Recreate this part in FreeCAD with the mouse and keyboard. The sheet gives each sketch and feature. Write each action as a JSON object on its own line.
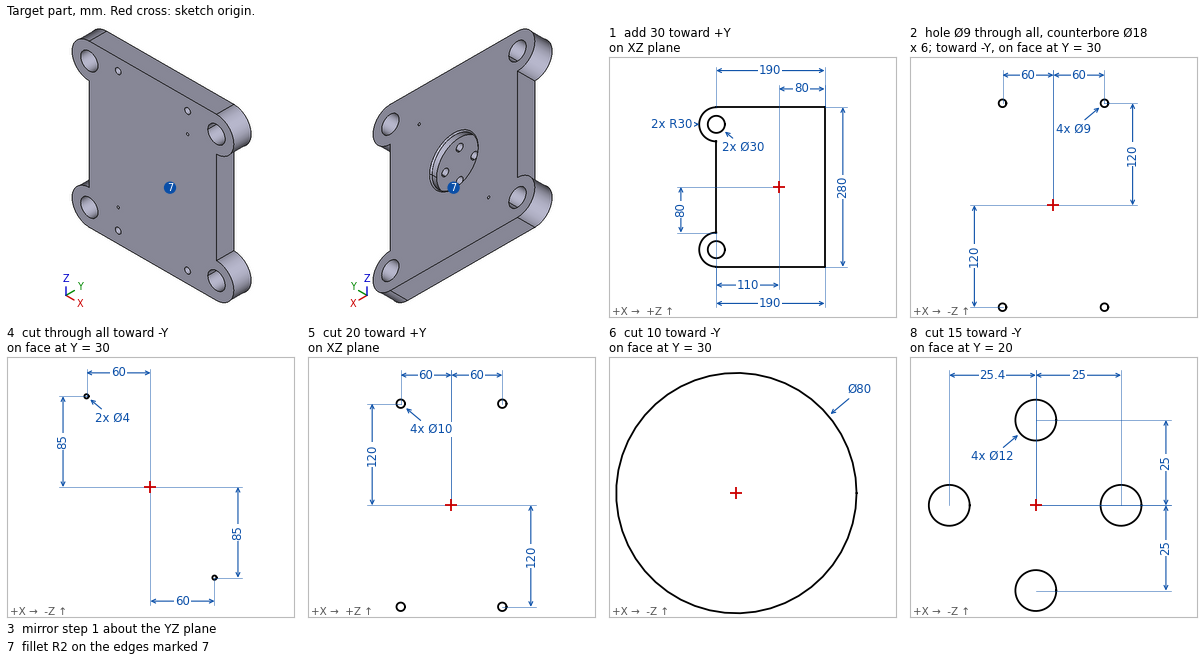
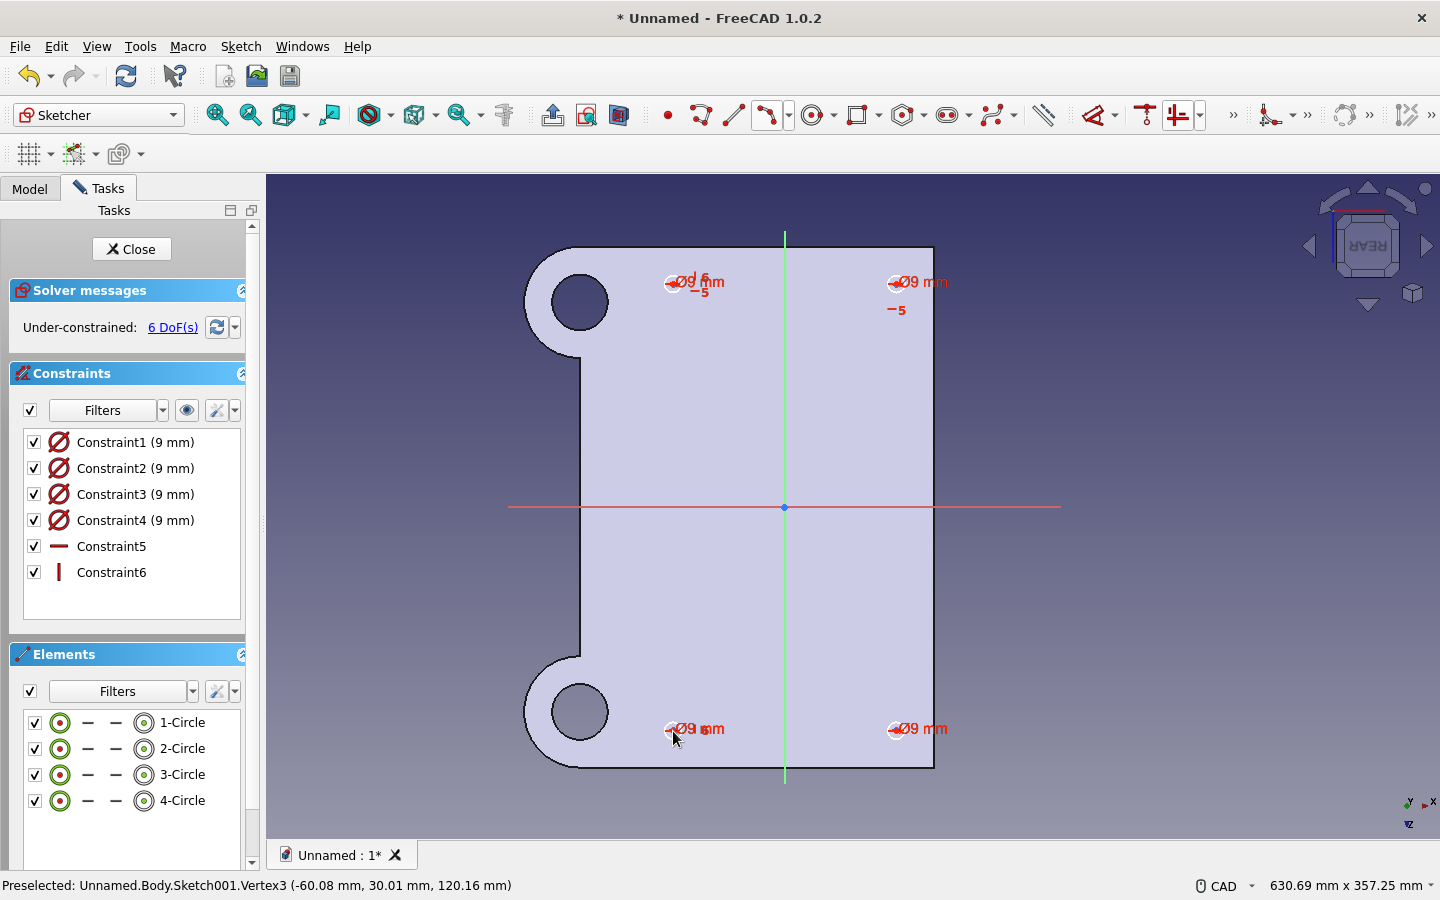
{"action": "left_click", "coordinate": [896, 284]}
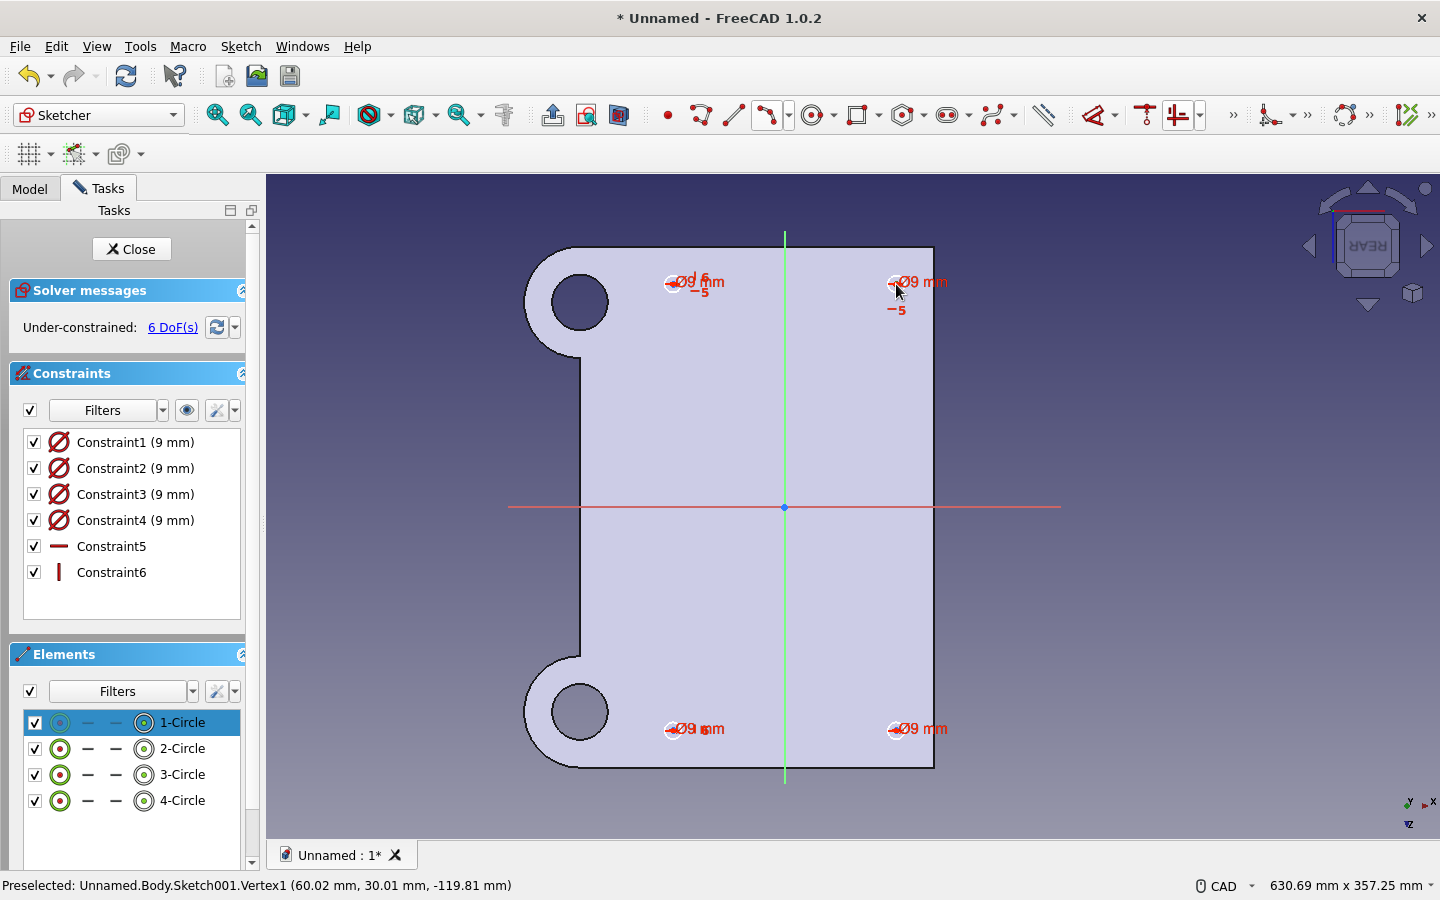
{"action": "left_click", "coordinate": [896, 731]}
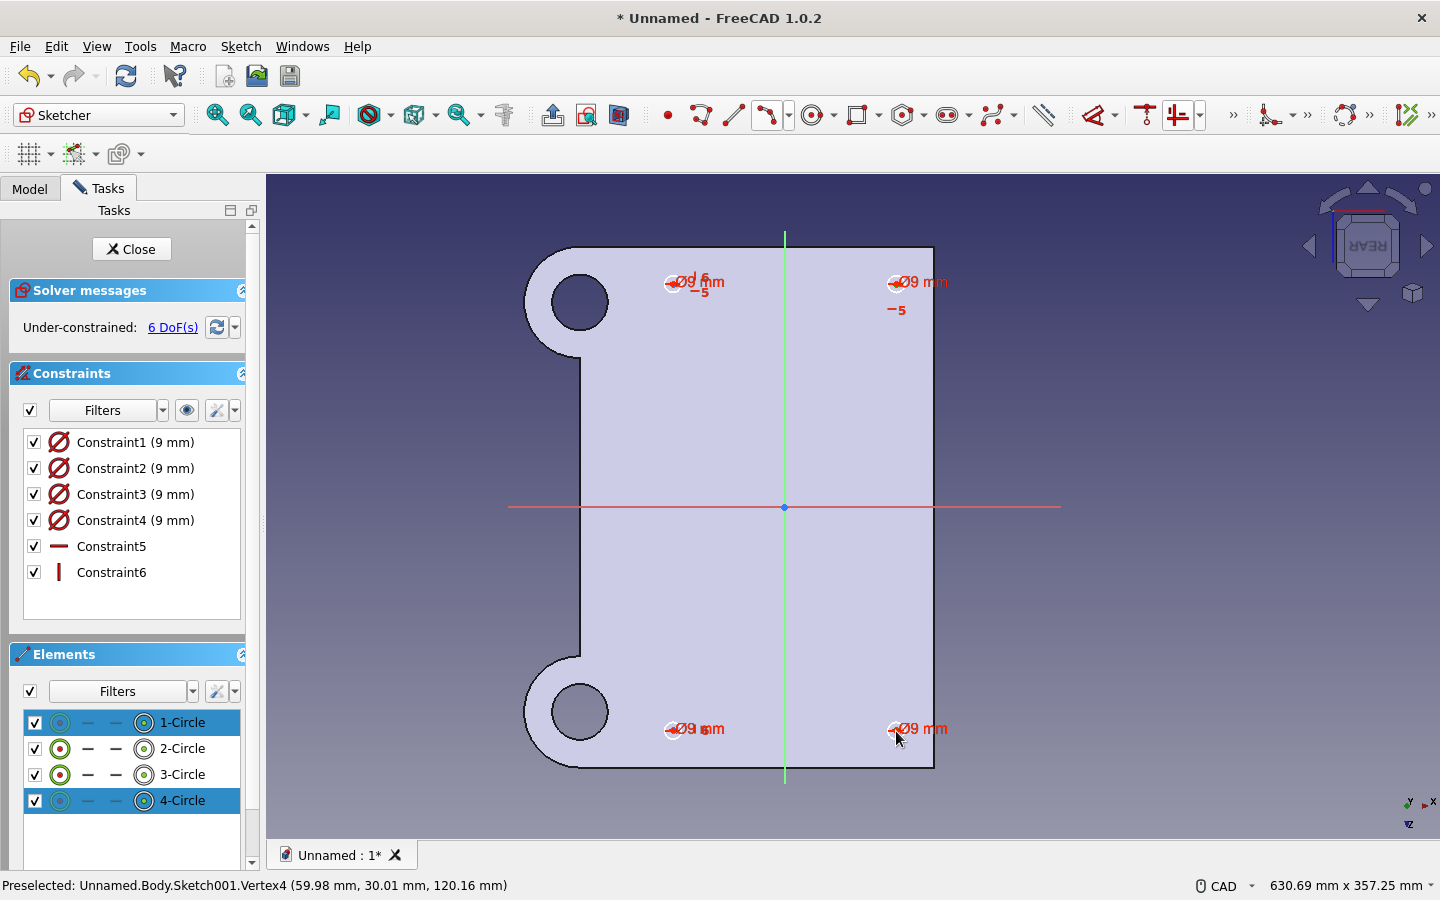
{"action": "left_click", "coordinate": [1200, 116]}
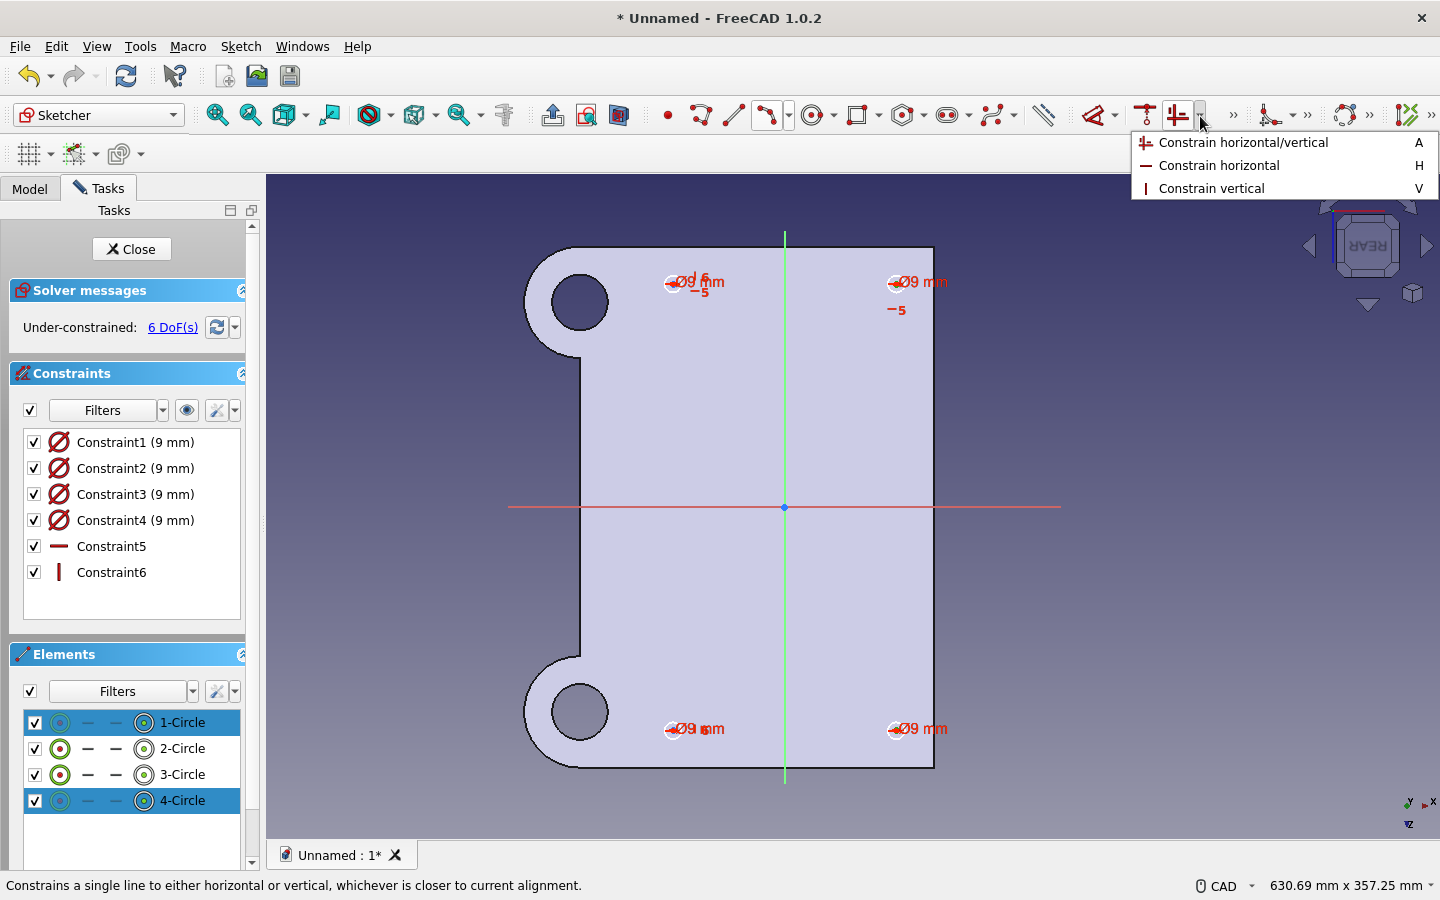
{"action": "left_click", "coordinate": [1285, 188]}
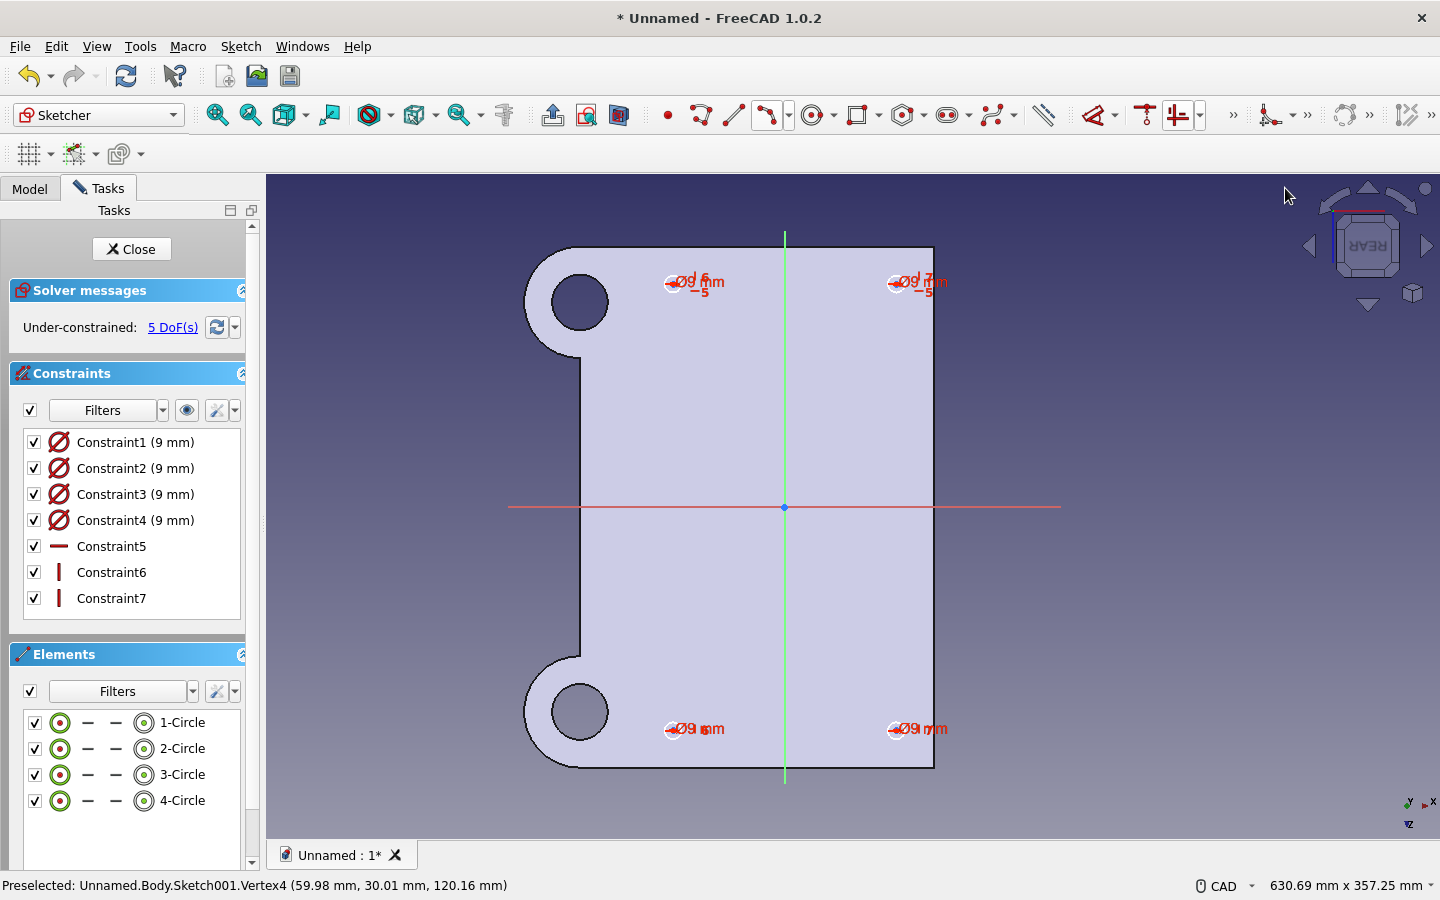
{"action": "left_click", "coordinate": [673, 731]}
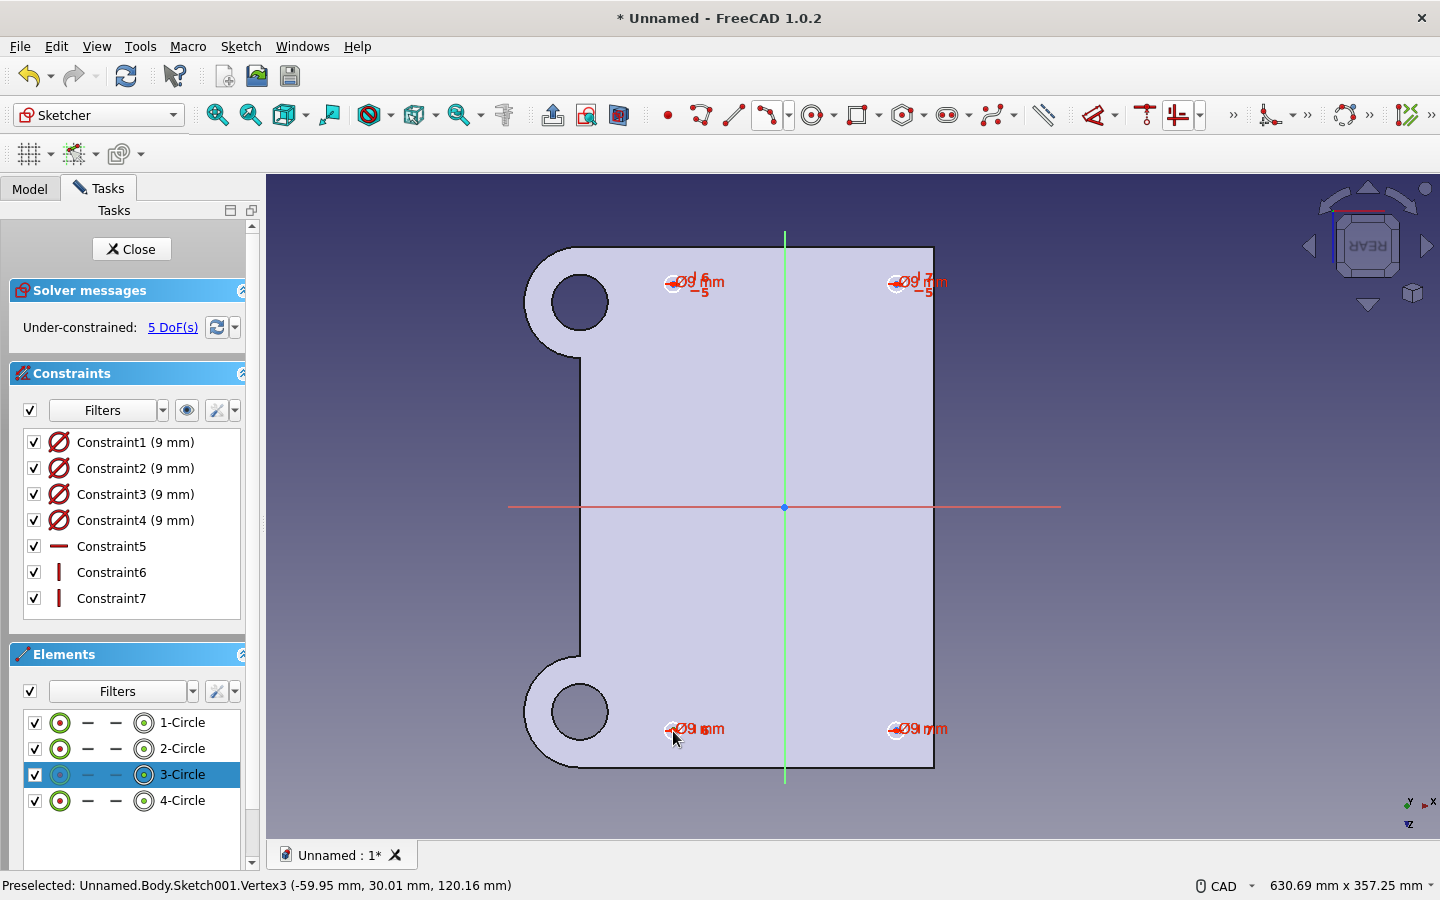
{"action": "left_click", "coordinate": [896, 731]}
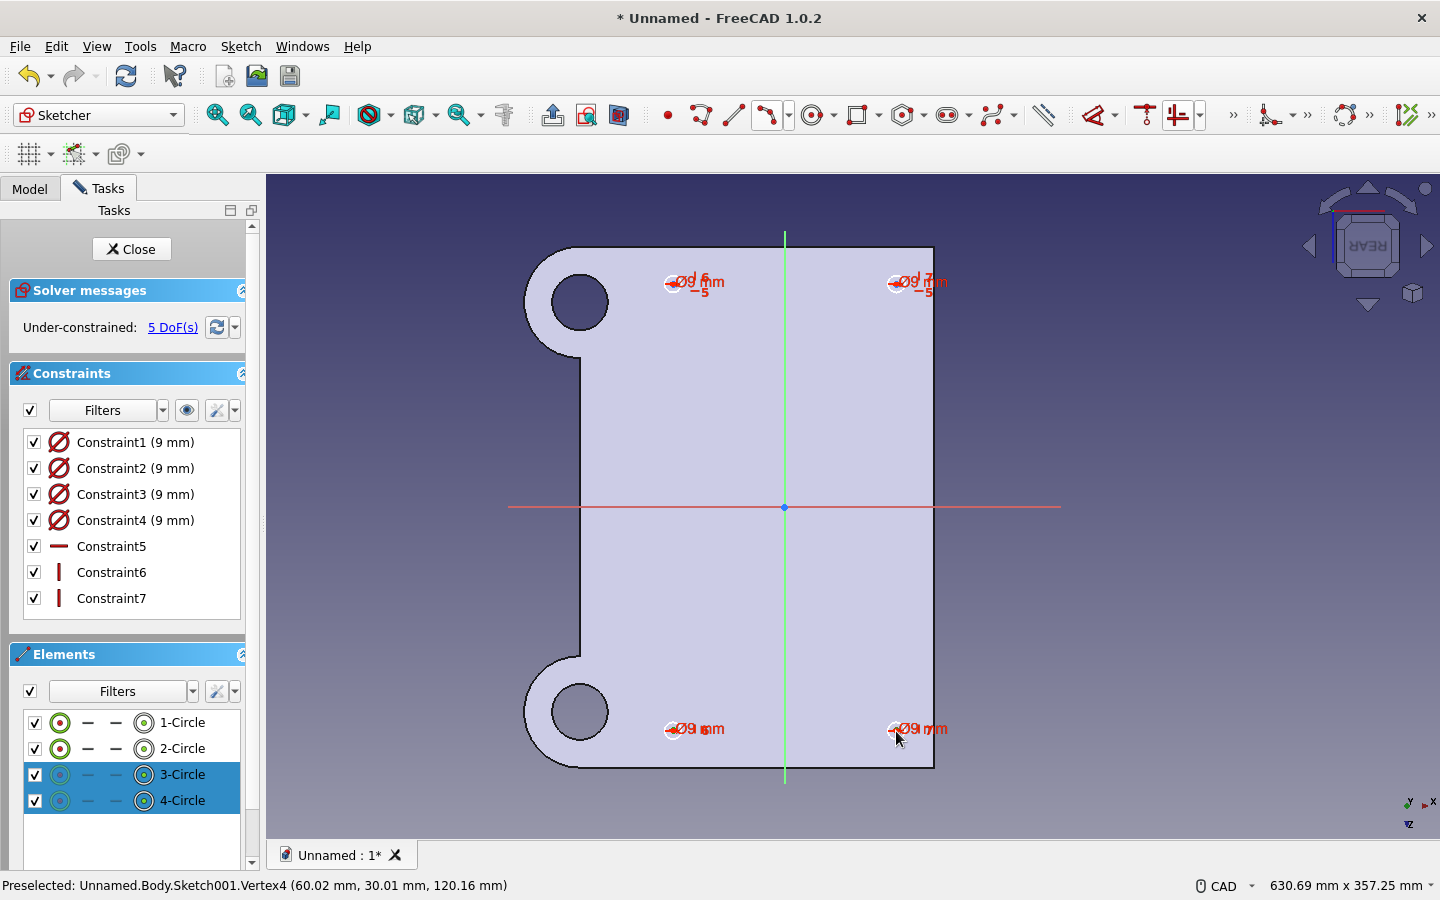
{"action": "left_click", "coordinate": [1200, 116]}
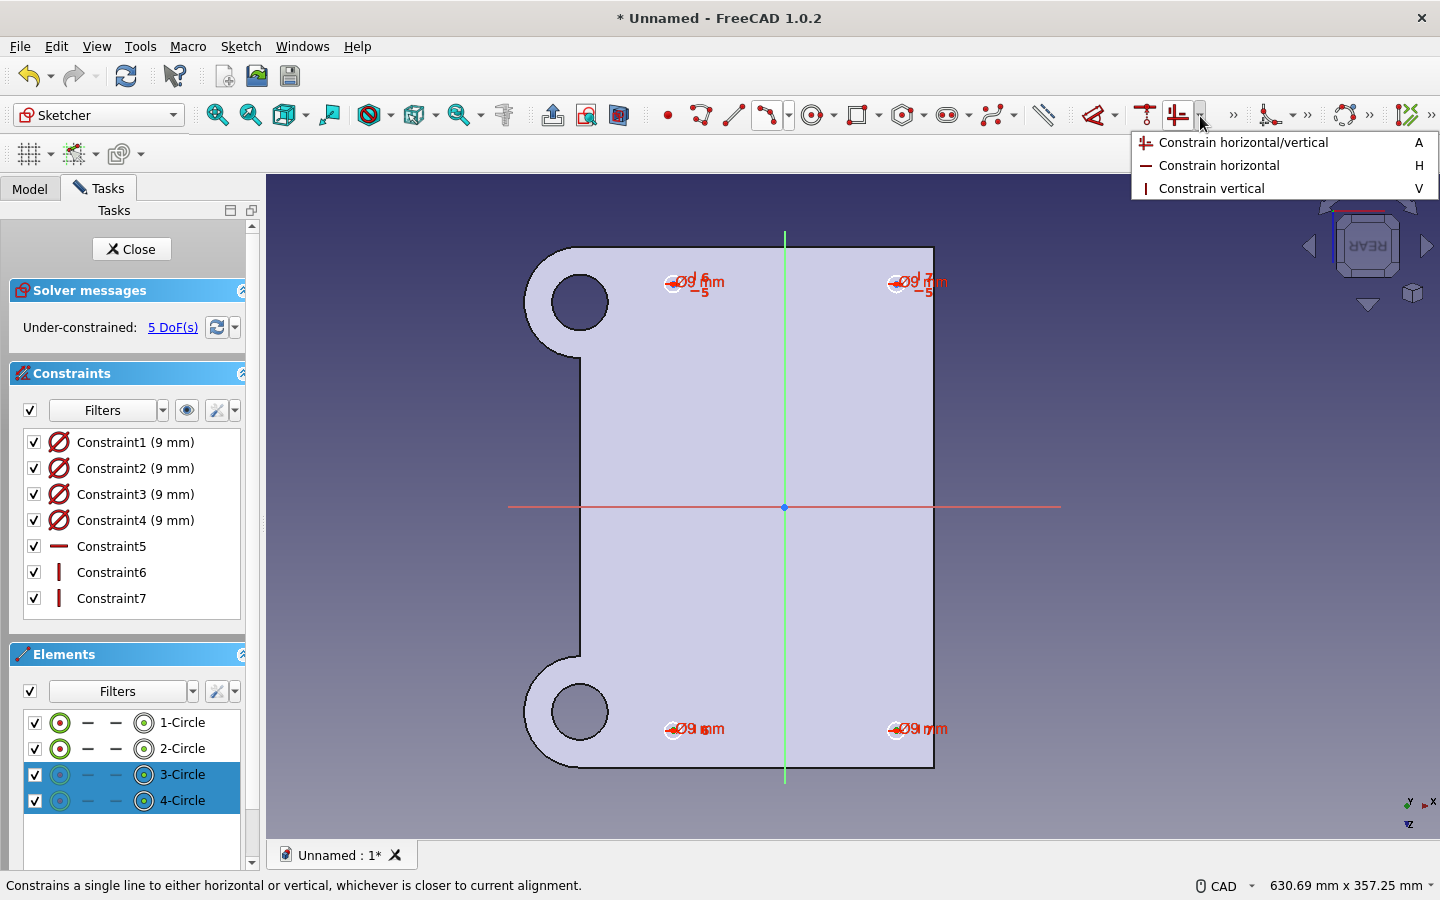
{"action": "left_click", "coordinate": [1285, 166]}